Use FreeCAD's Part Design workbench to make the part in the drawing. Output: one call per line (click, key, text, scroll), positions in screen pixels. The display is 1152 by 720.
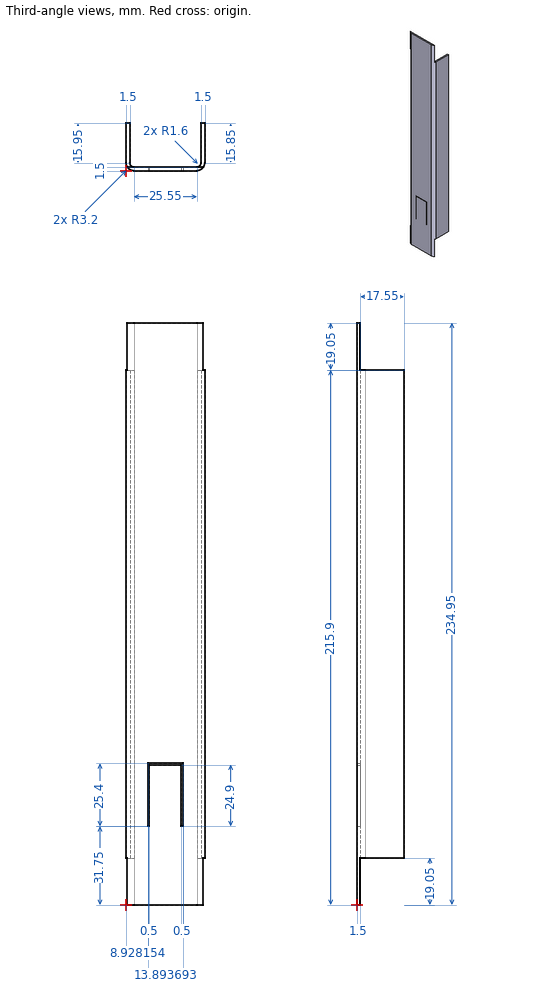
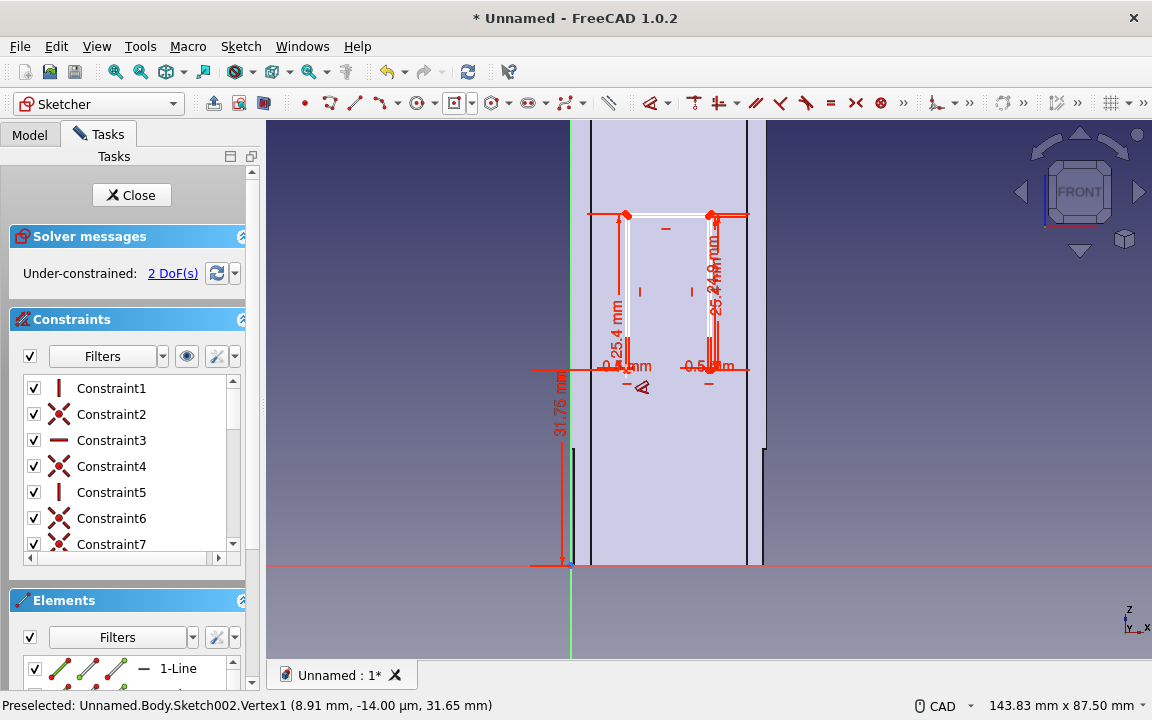
scroll(651, 214, up, 8)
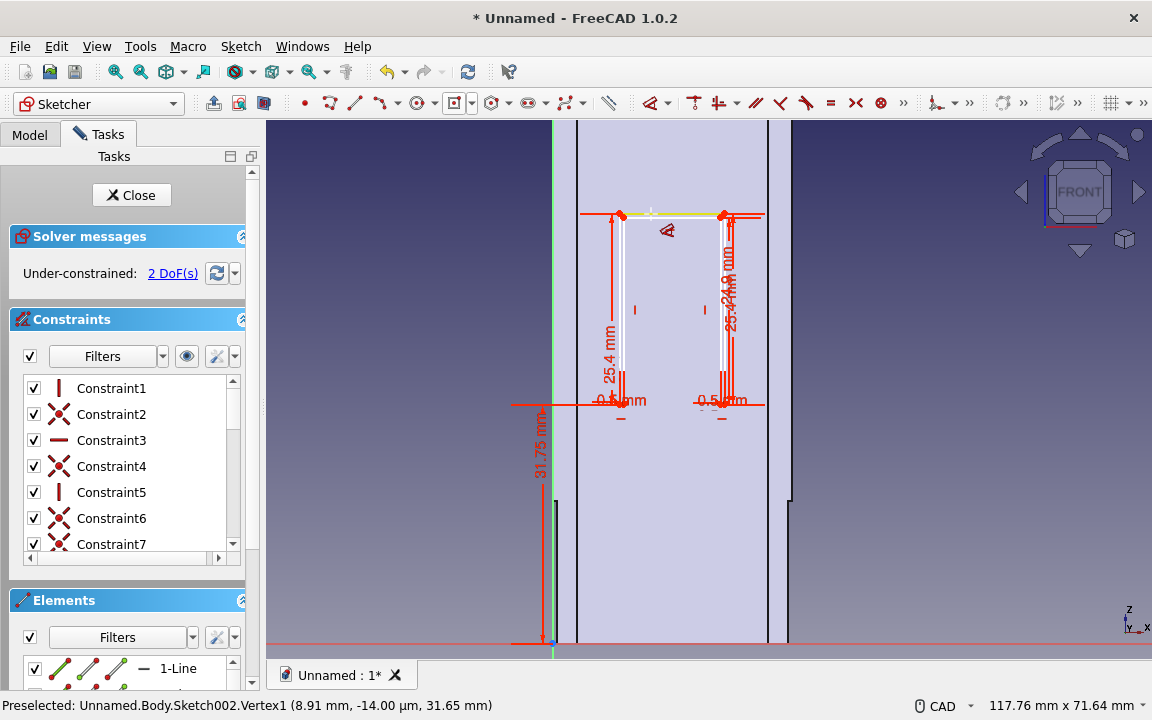
click(651, 213)
click(736, 179)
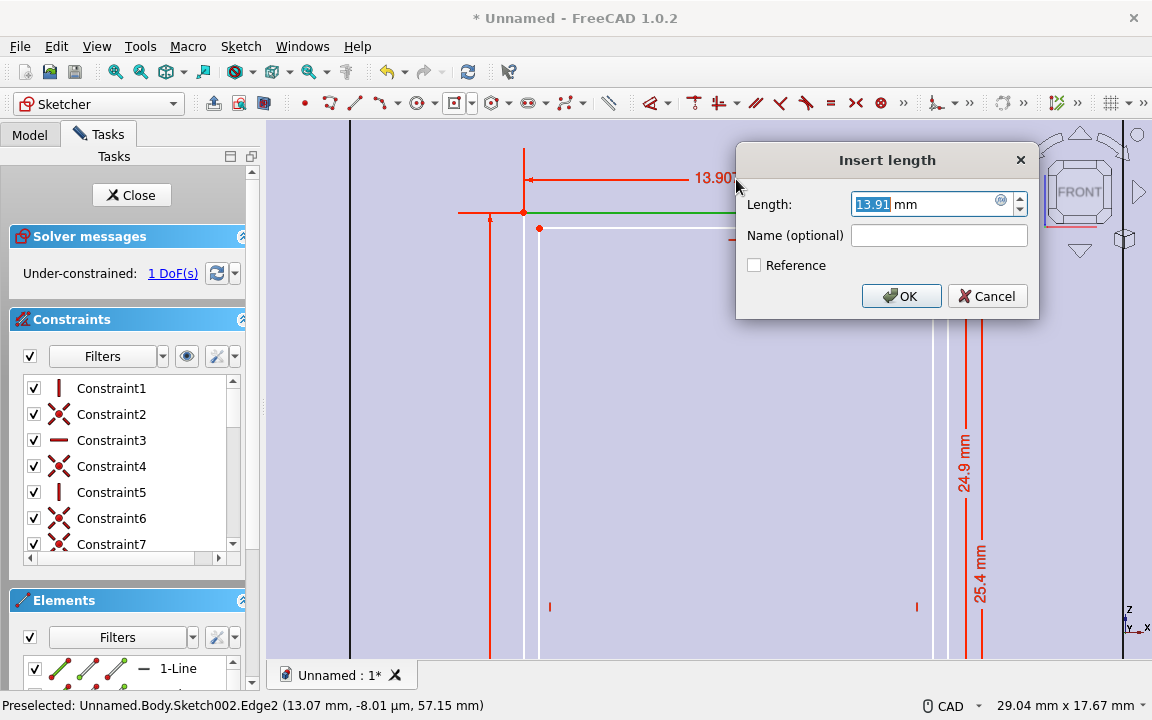
text(13.893693)
key(Return)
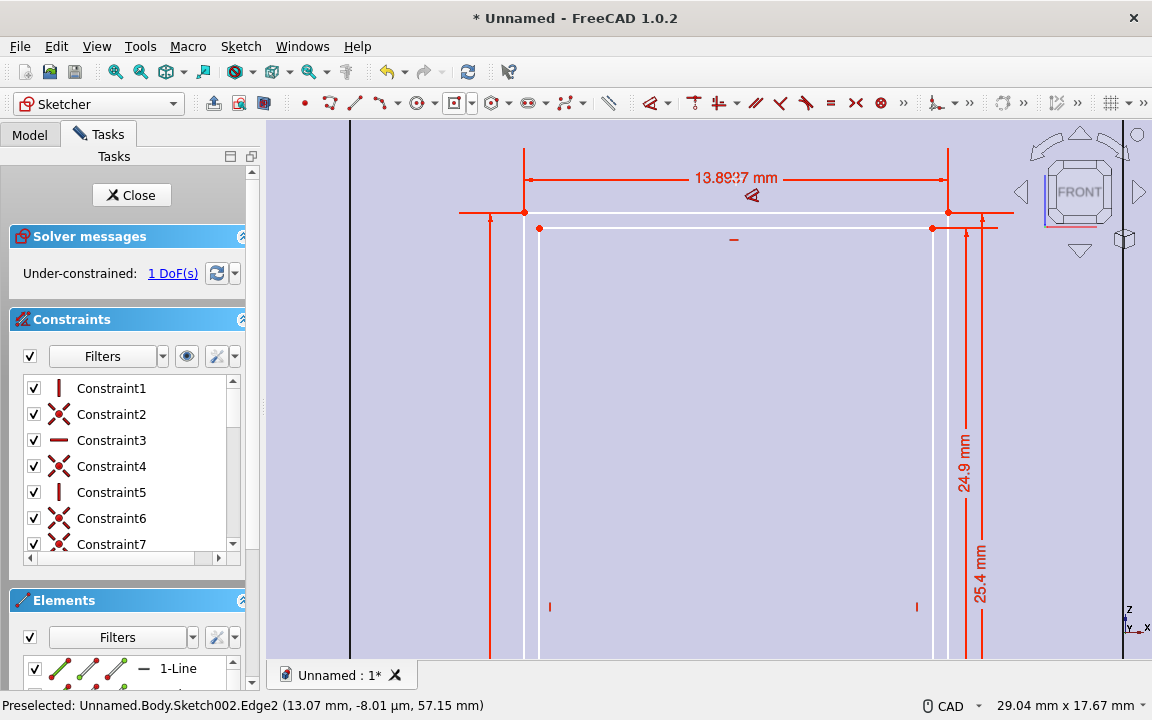
scroll(651, 214, down, 8)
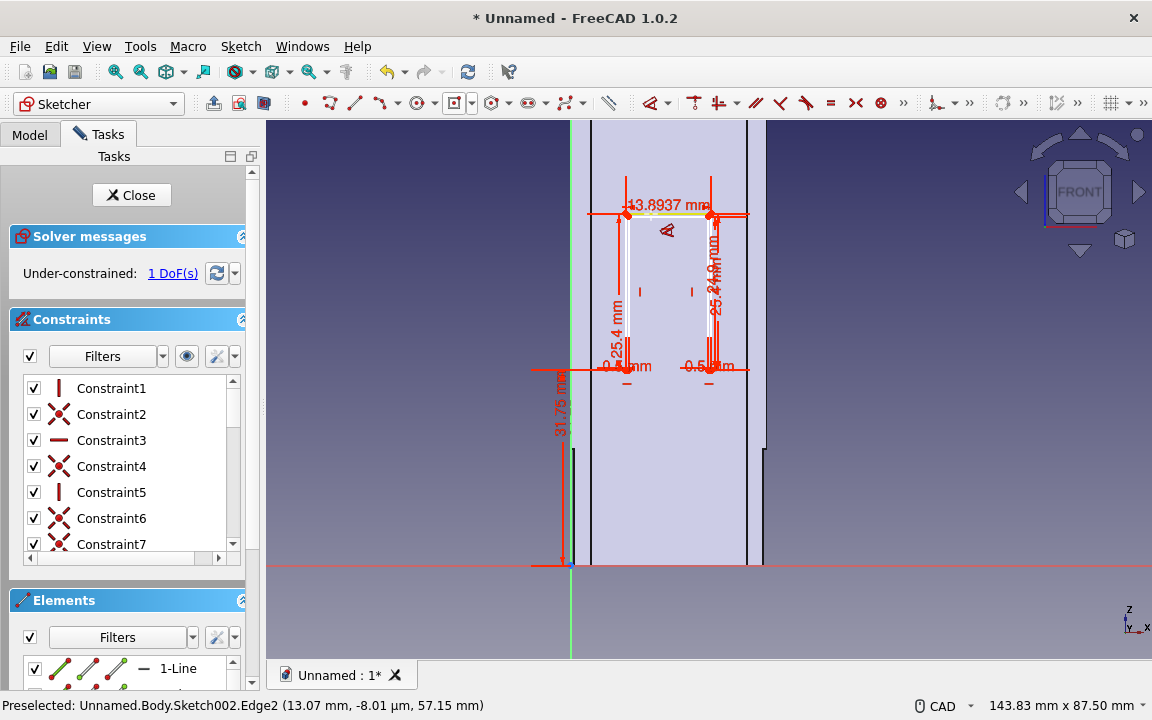
scroll(626, 370, up, 7)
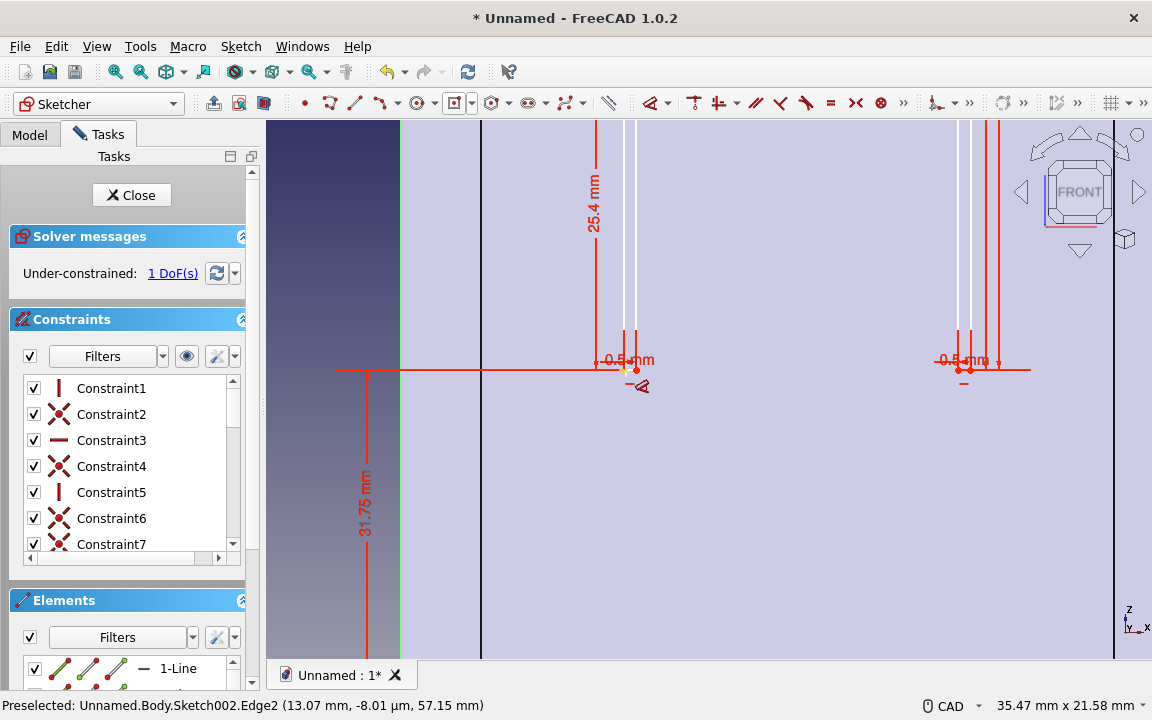
click(624, 370)
click(512, 336)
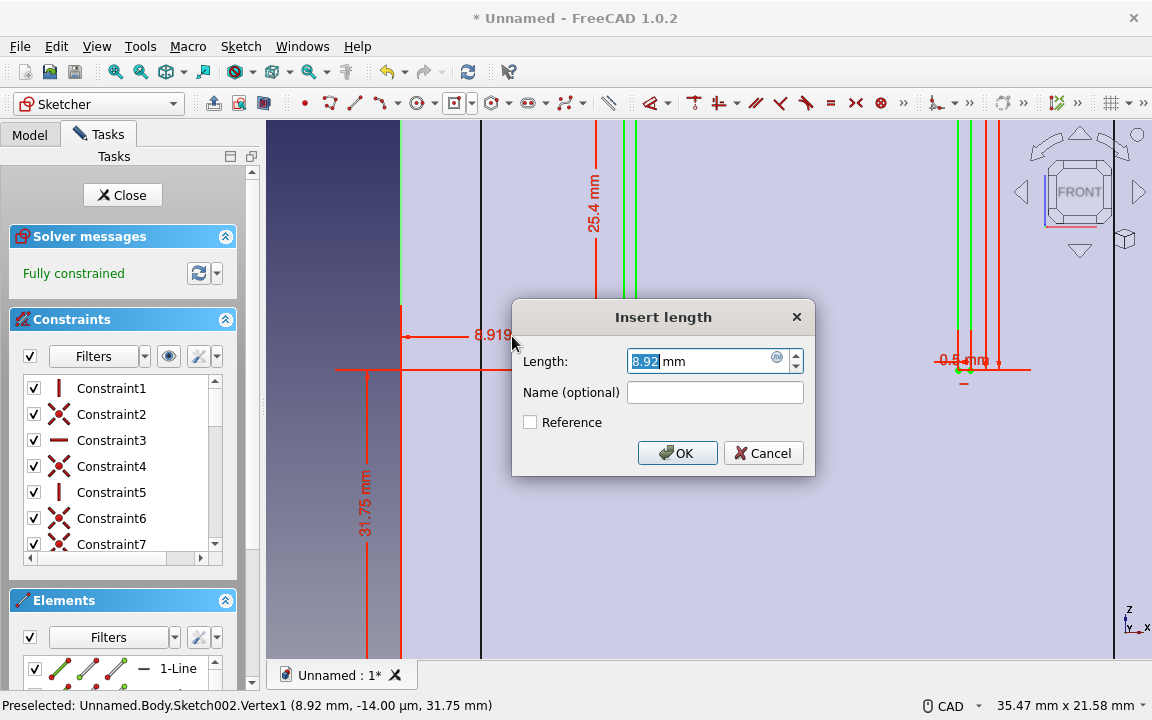
text(8.928154)
key(Return)
key(Escape)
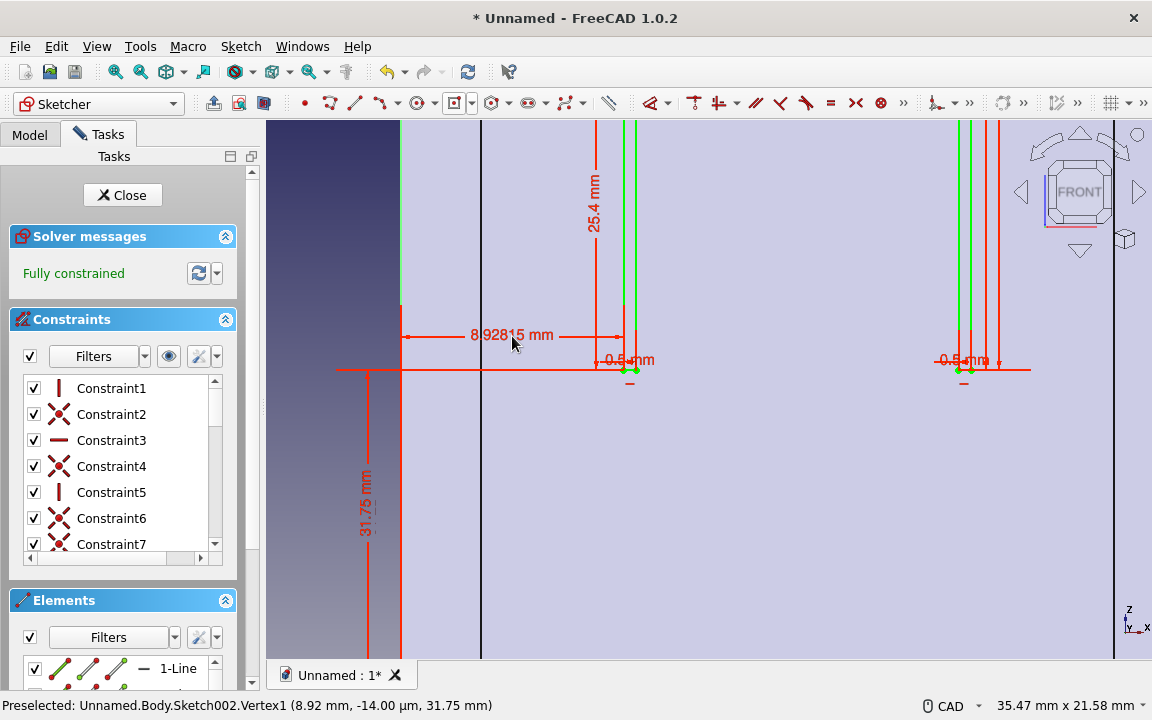
click(123, 195)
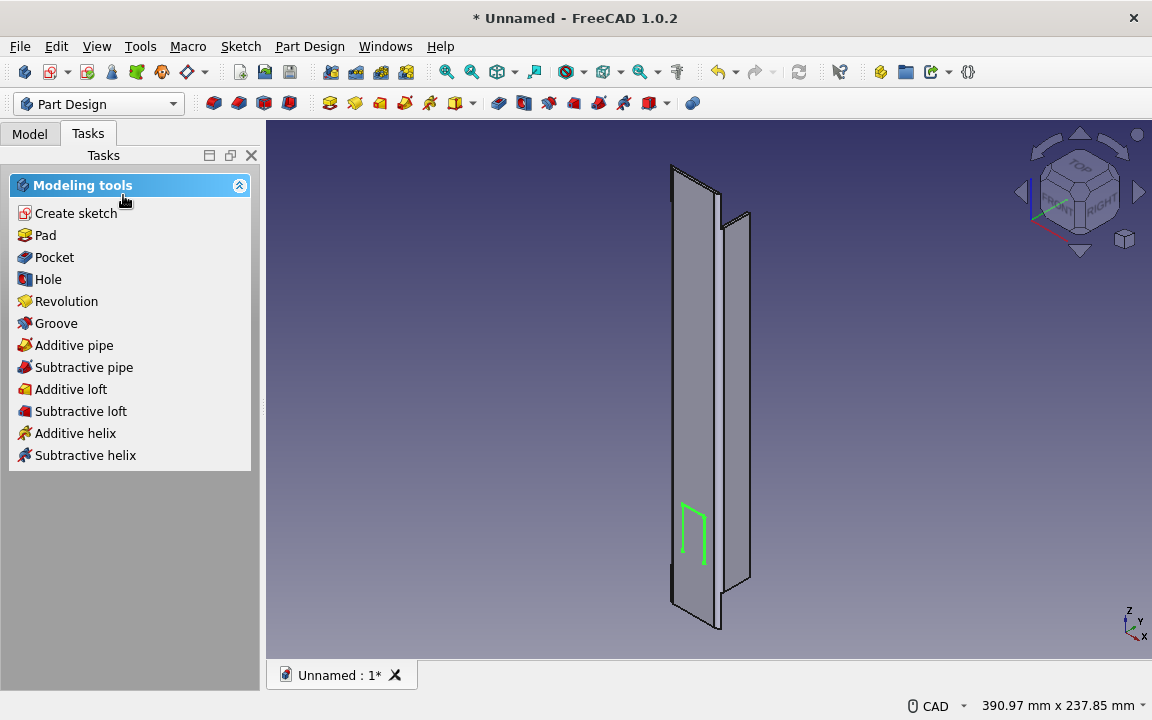
click(499, 104)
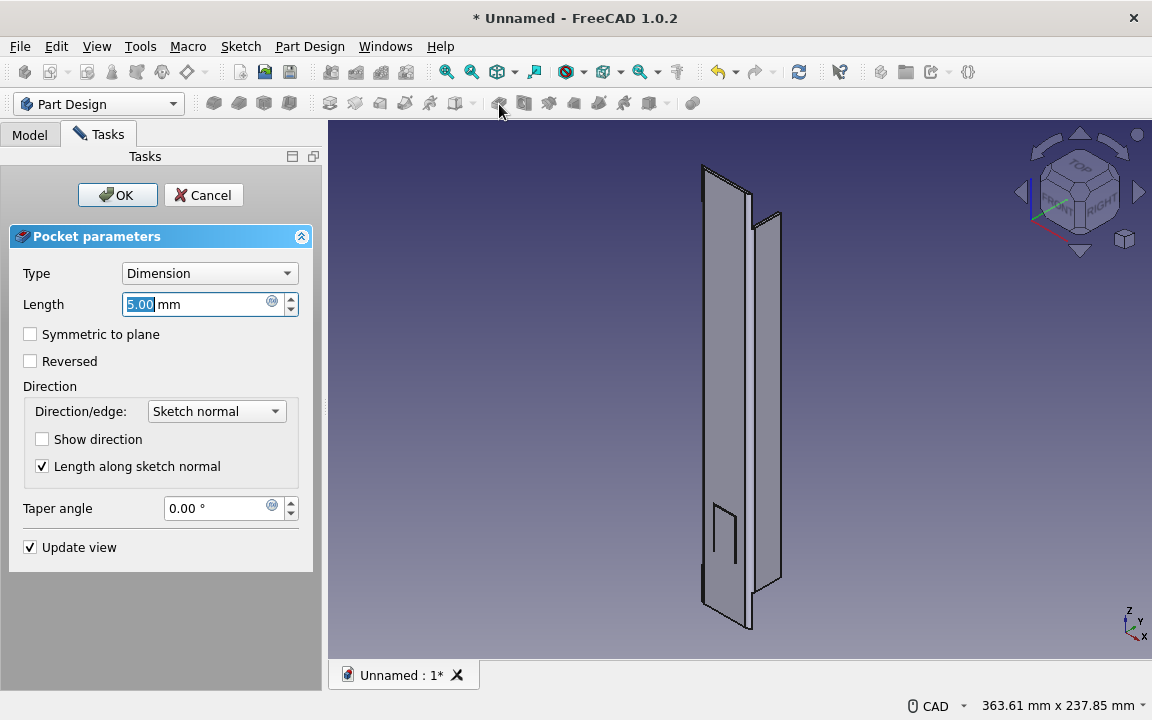
click(210, 274)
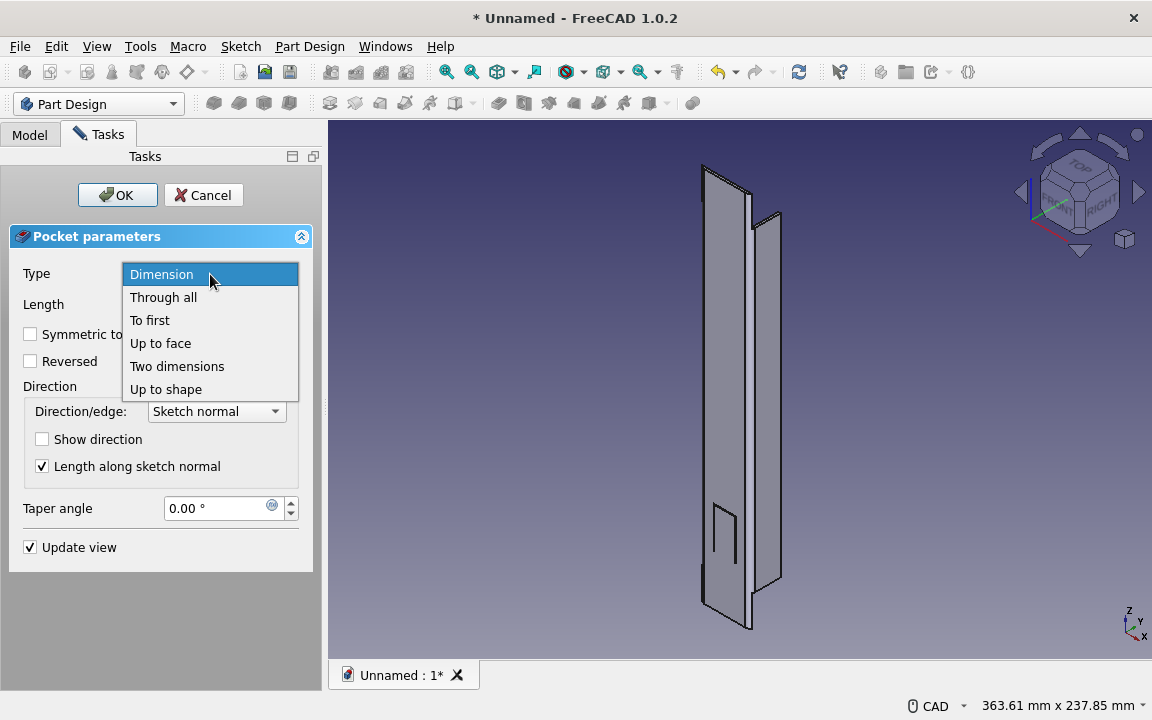
click(208, 298)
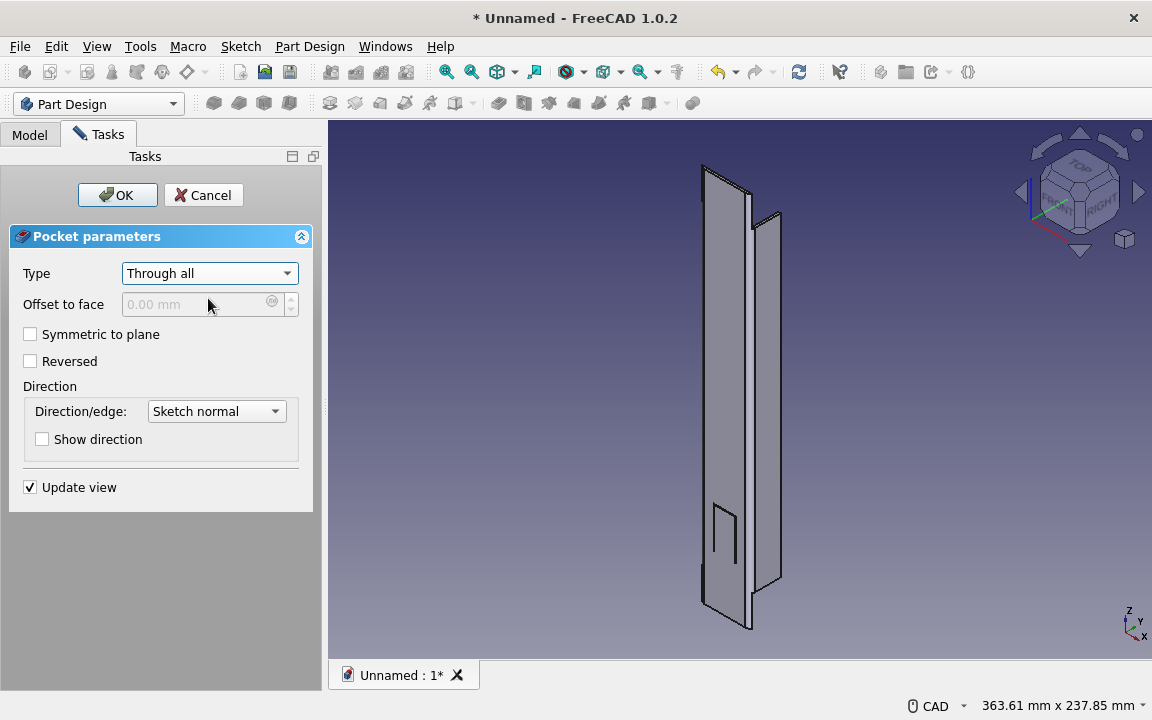
click(118, 195)